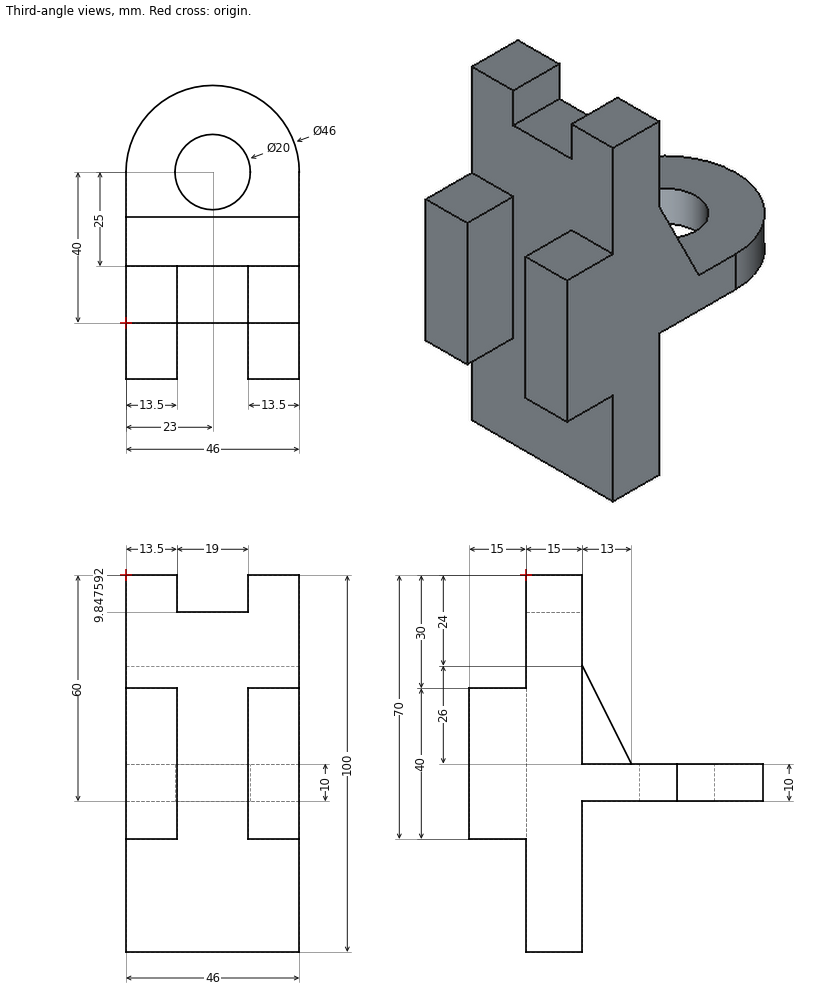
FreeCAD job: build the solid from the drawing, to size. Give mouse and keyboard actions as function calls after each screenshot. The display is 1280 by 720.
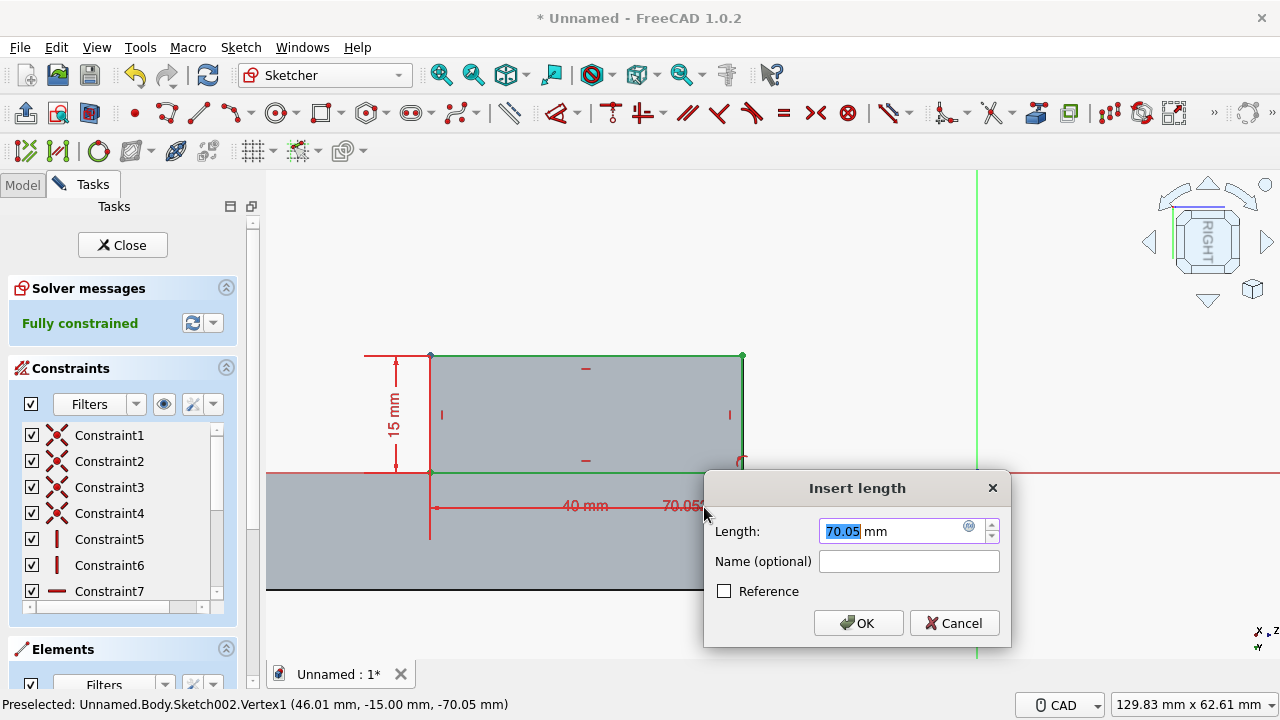
text(70)
key(Return)
key(Escape)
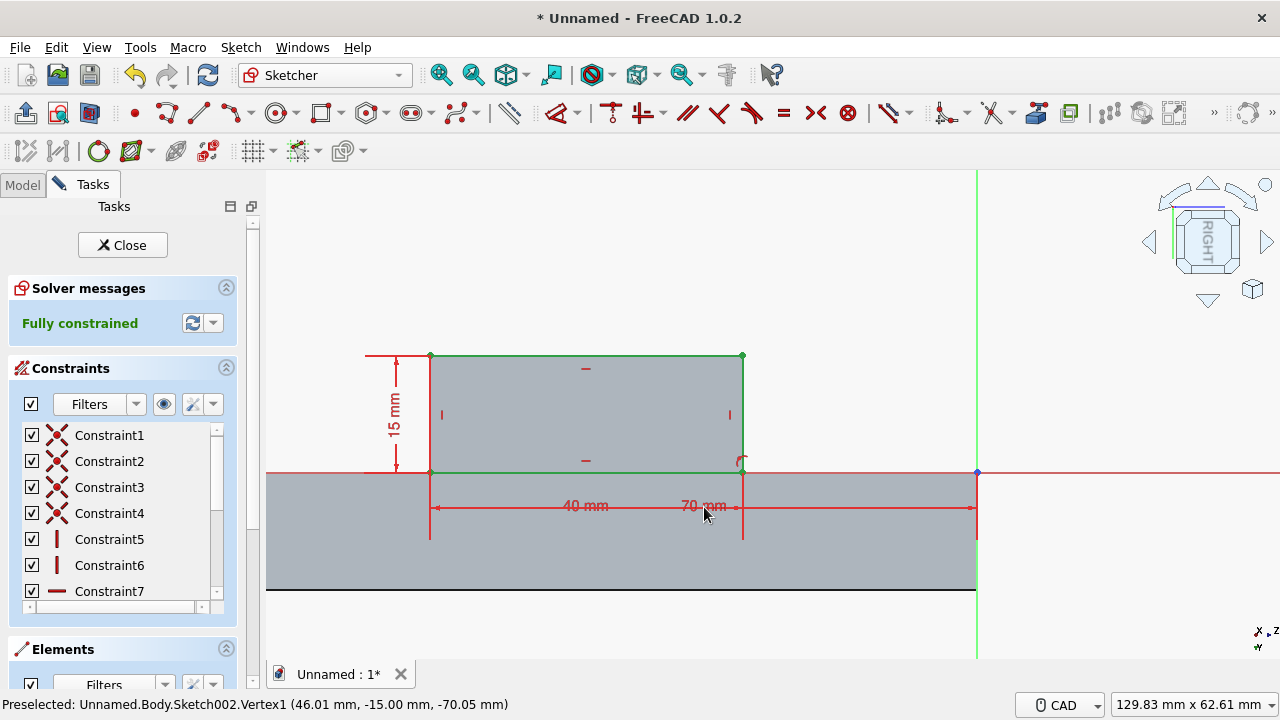
click(123, 245)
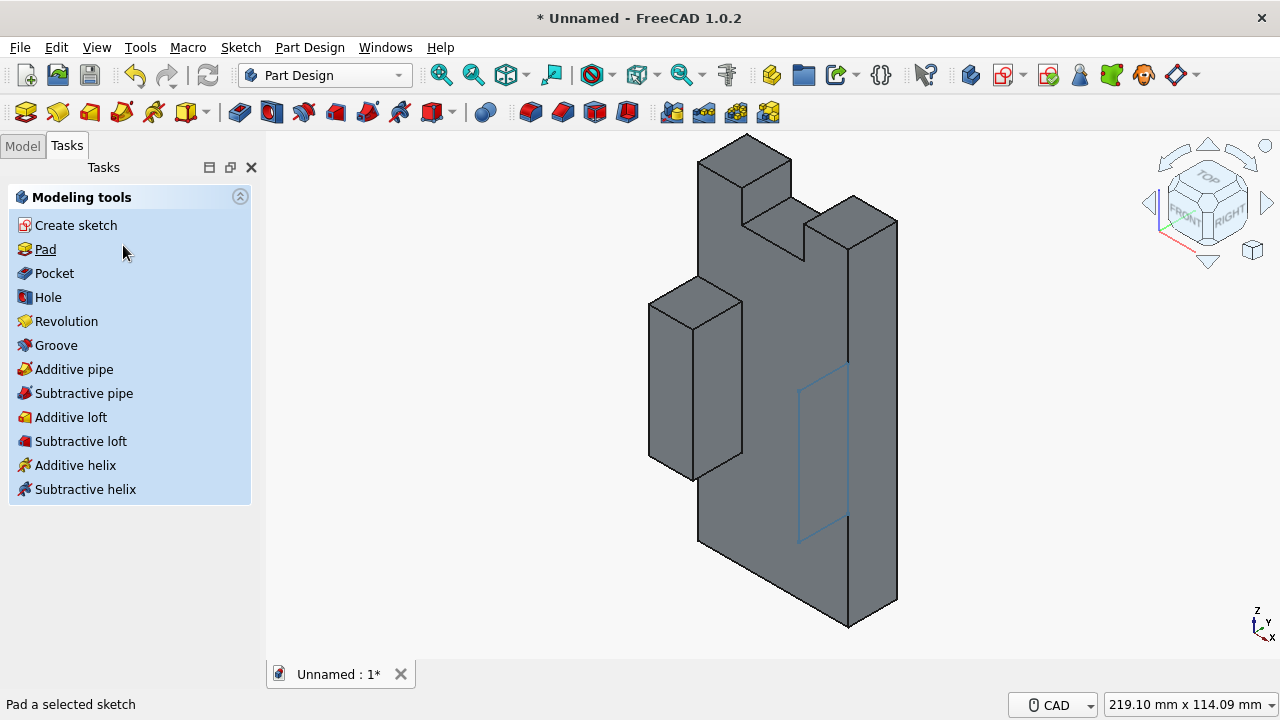
click(26, 112)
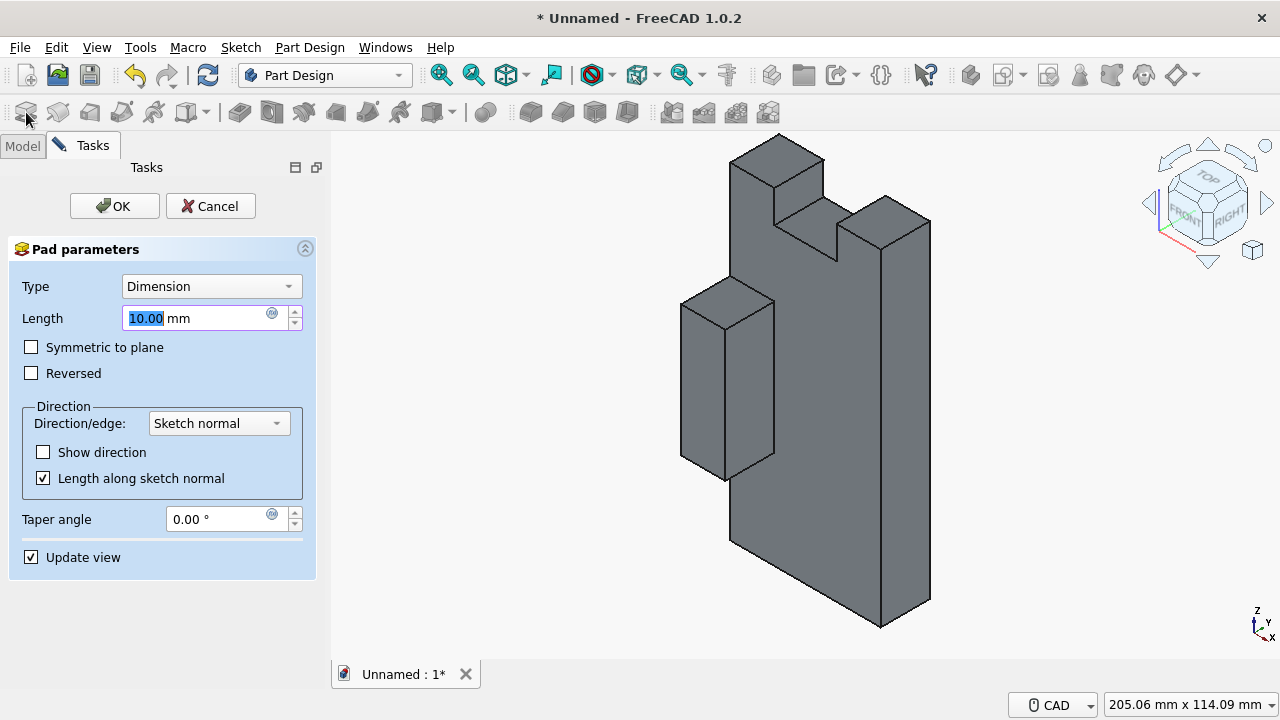
text(13.5)
key(Tab)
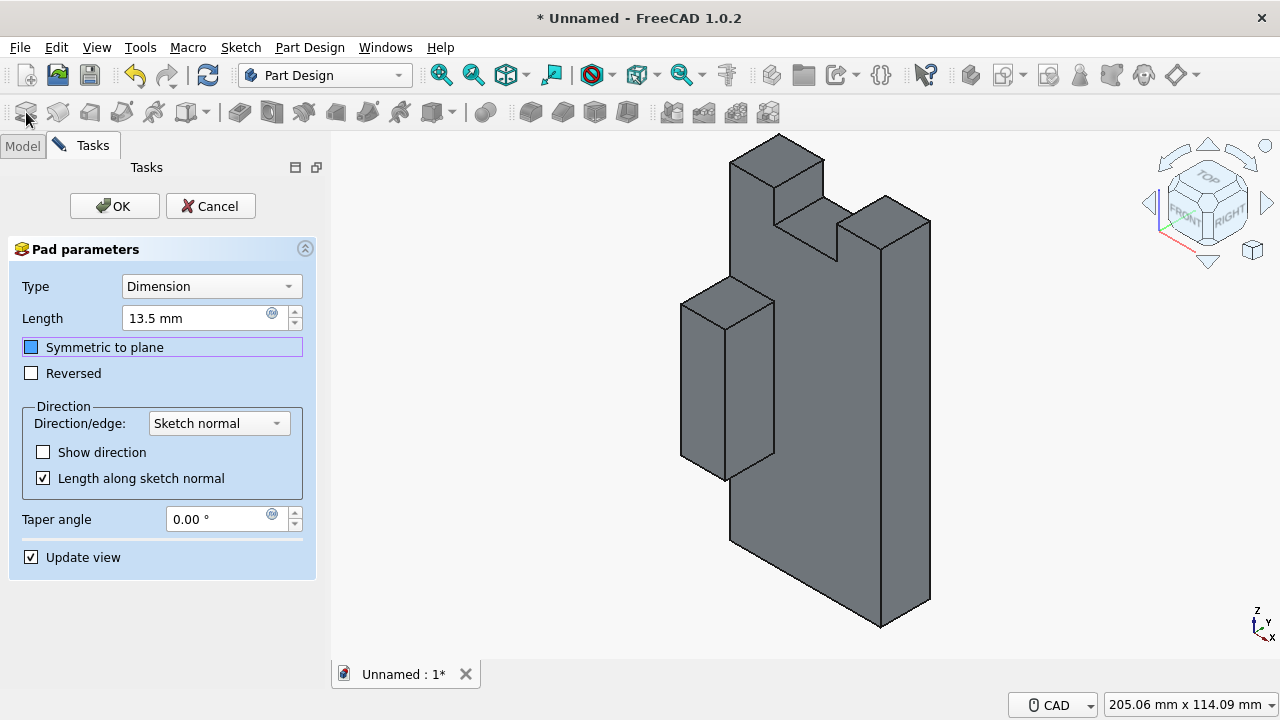
click(30, 373)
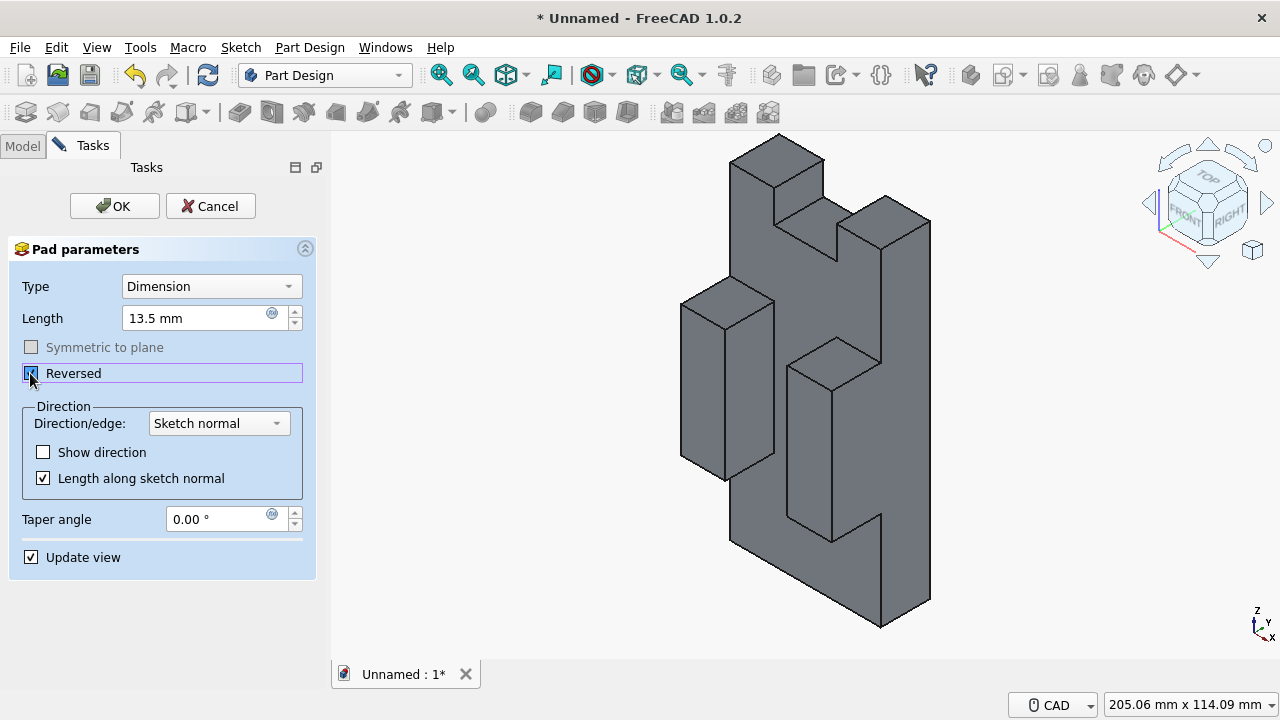
click(115, 206)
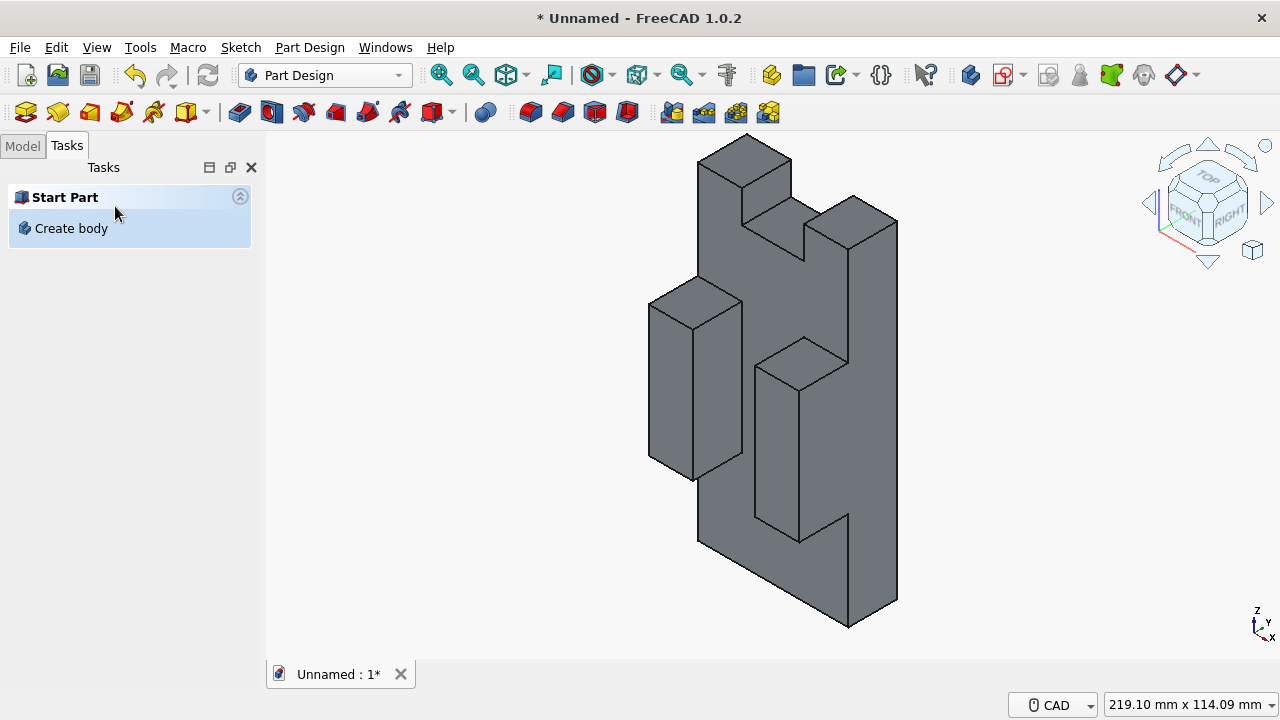
key(4)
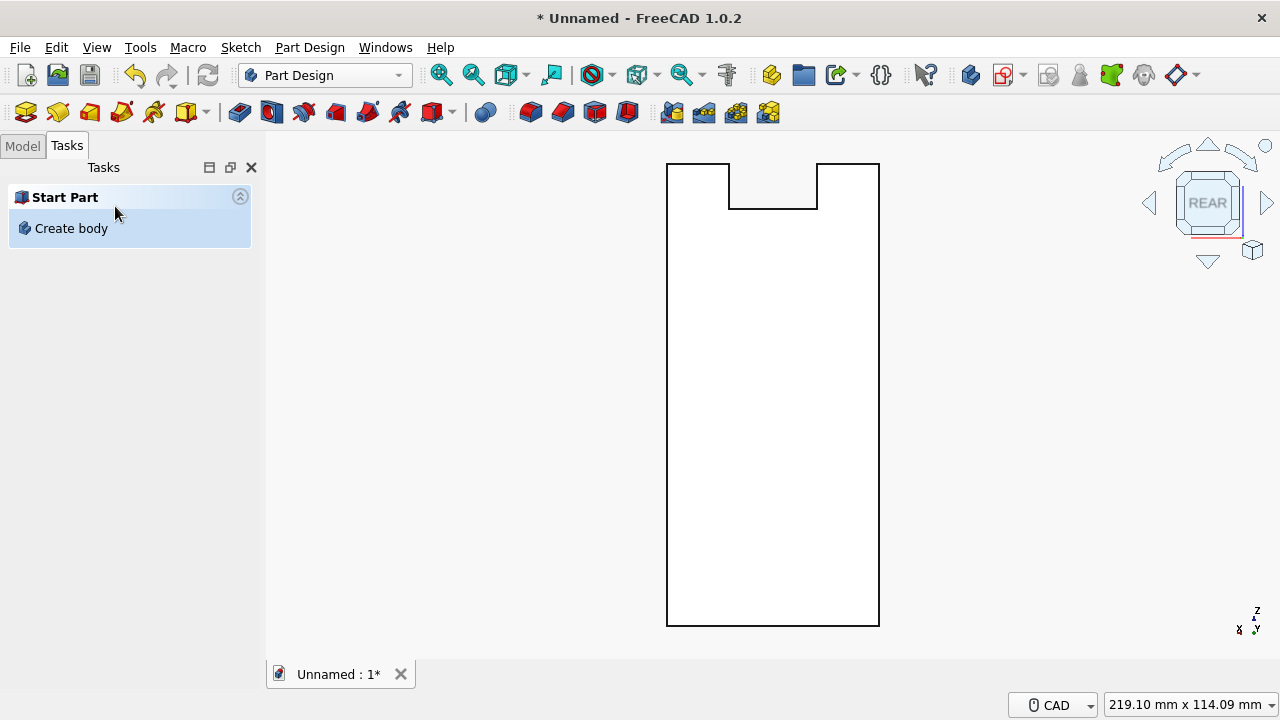
click(773, 328)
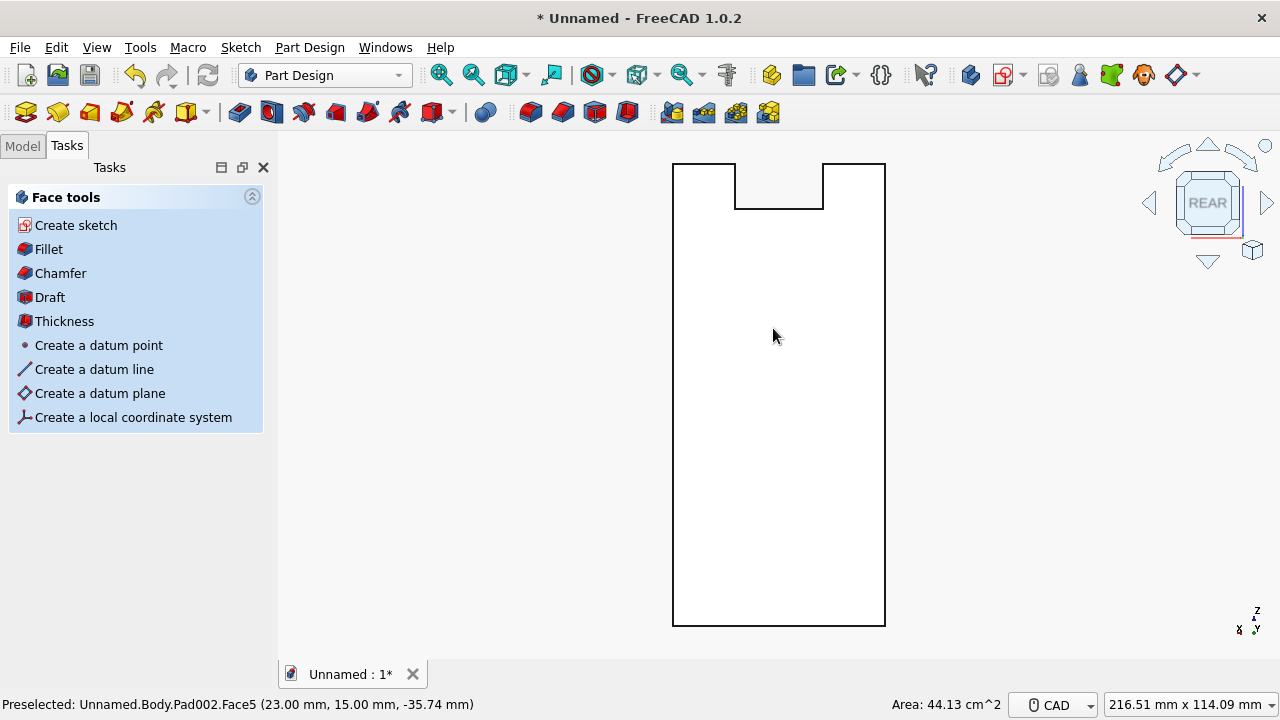
click(1004, 76)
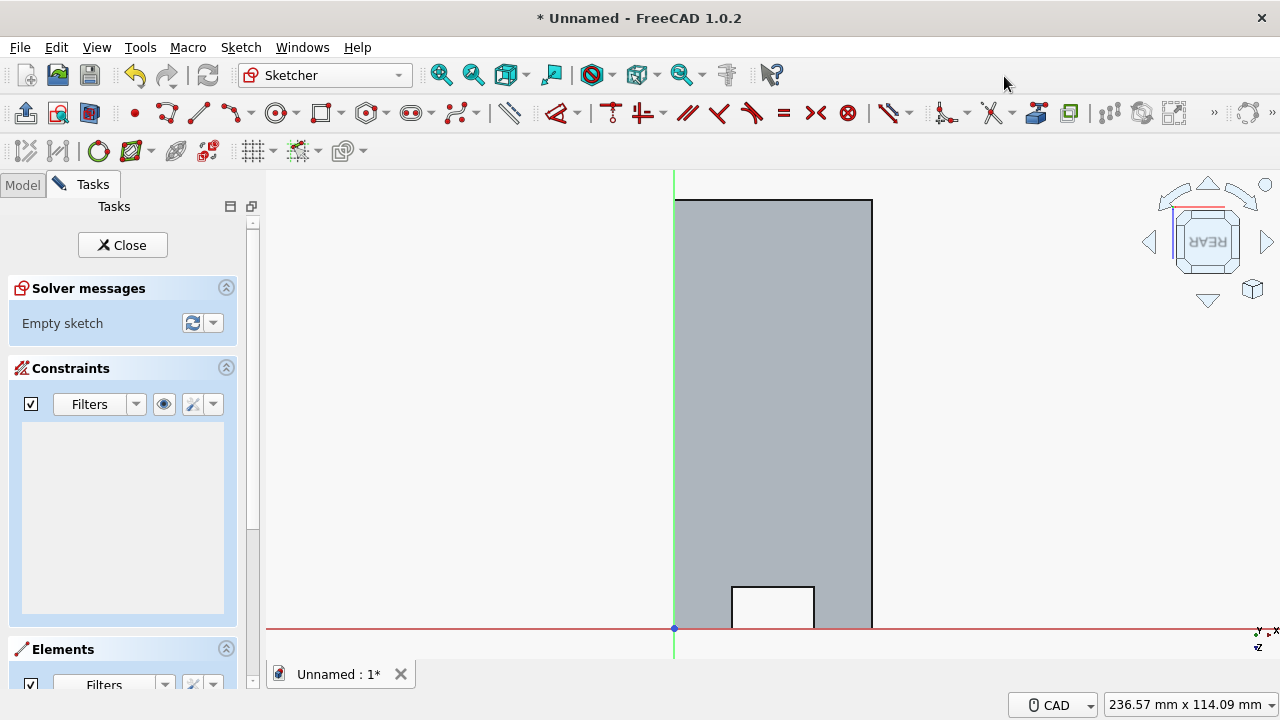
scroll(395, 198, down, 1)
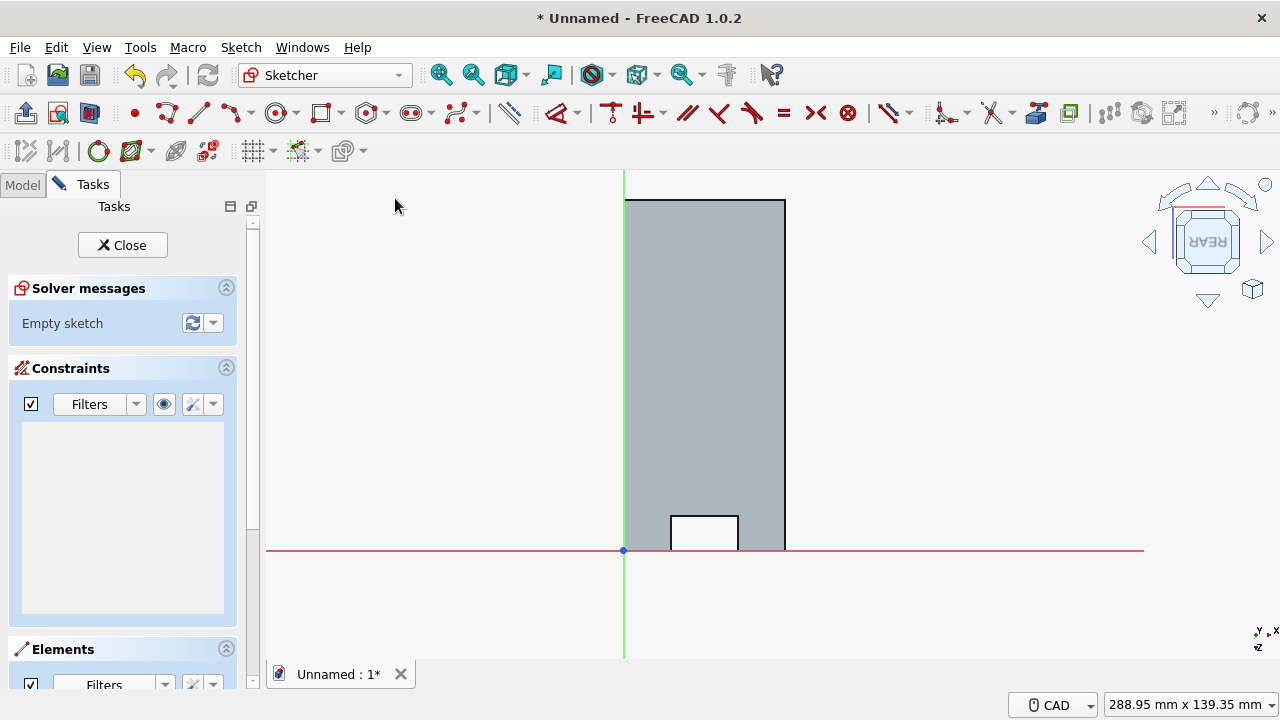
scroll(705, 508, up, 2)